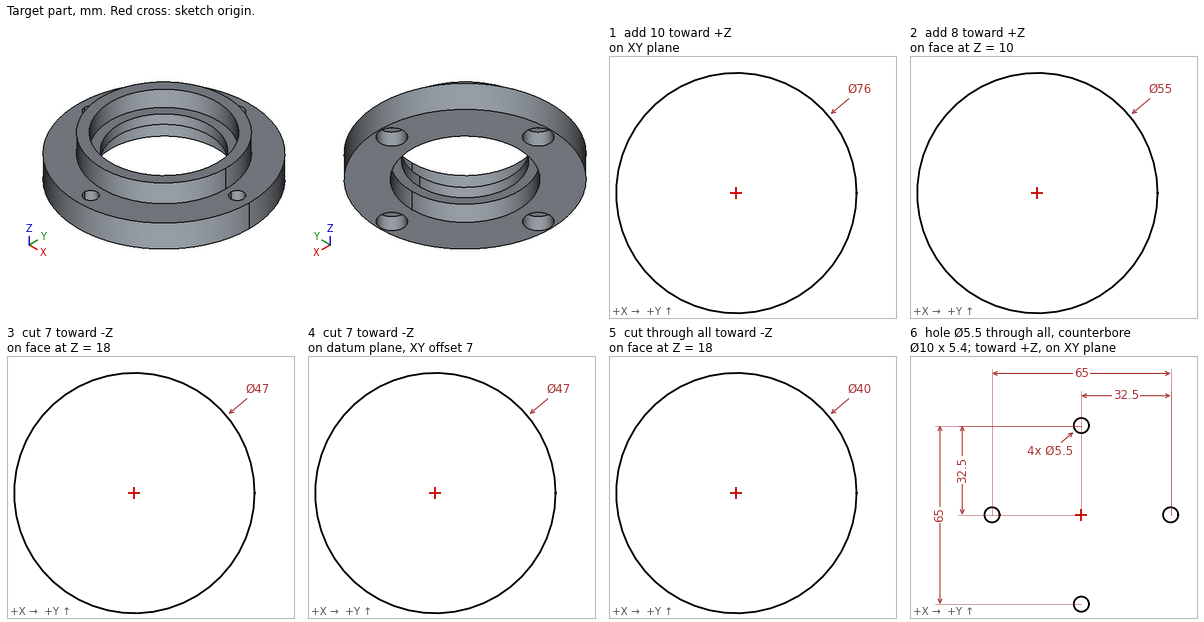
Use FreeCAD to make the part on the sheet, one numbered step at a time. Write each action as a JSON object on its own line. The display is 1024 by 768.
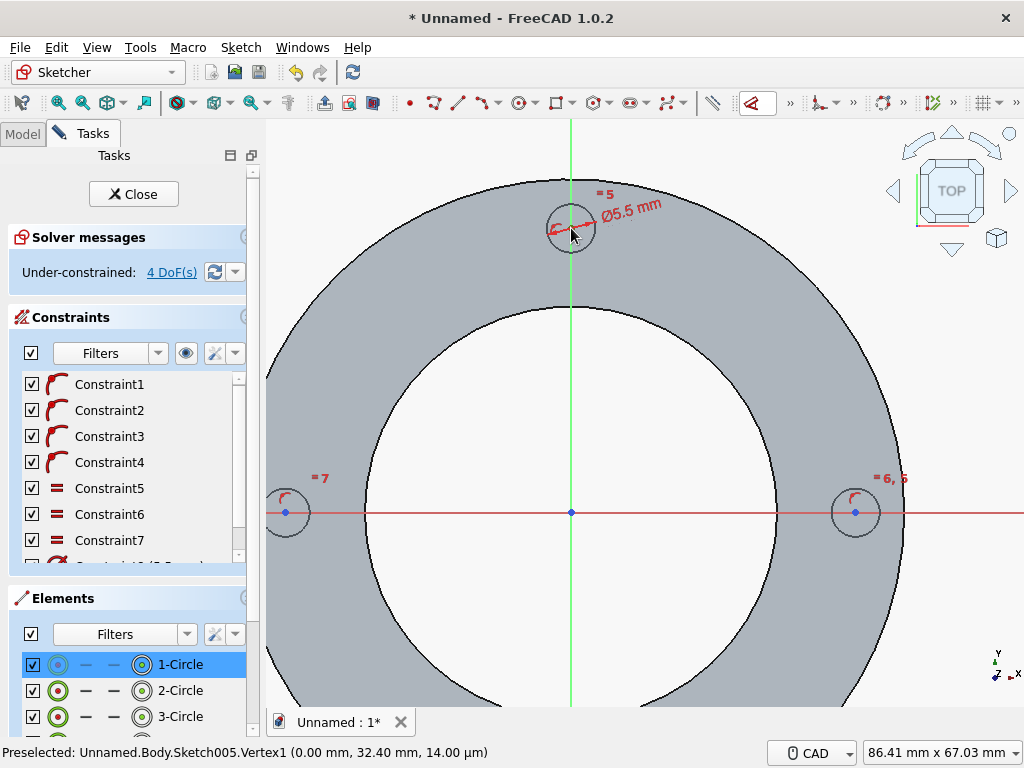
{"action": "scroll", "coordinate": [588, 210], "scroll_direction": "down", "scroll_amount": 2}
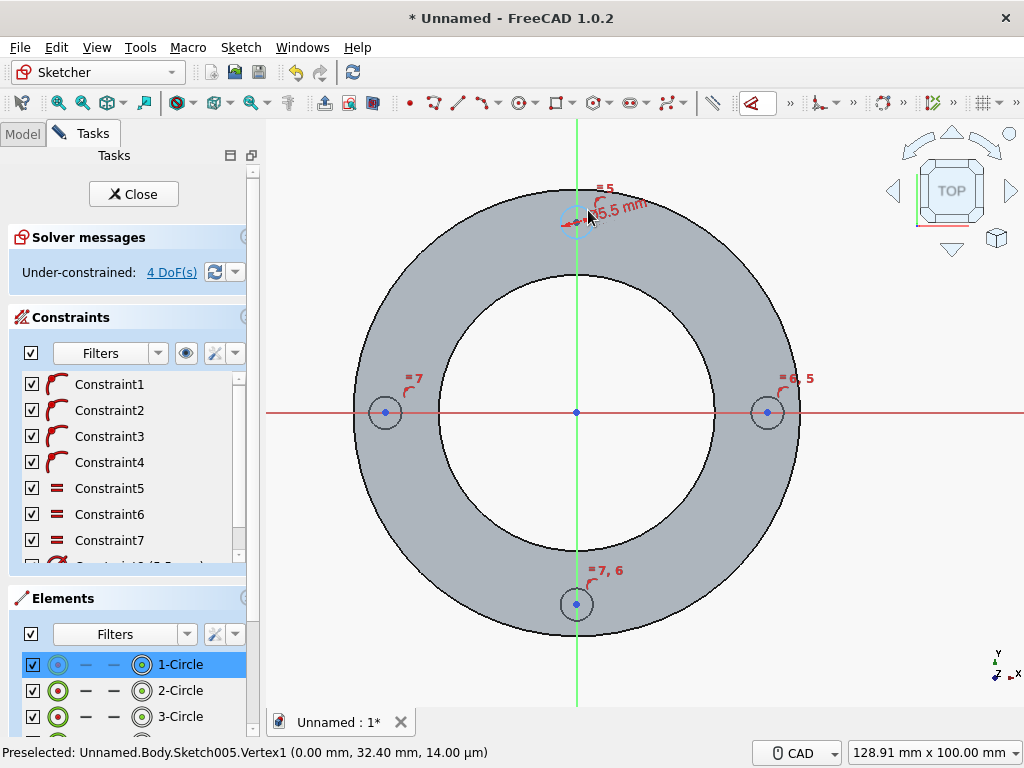
{"action": "left_click", "coordinate": [577, 605]}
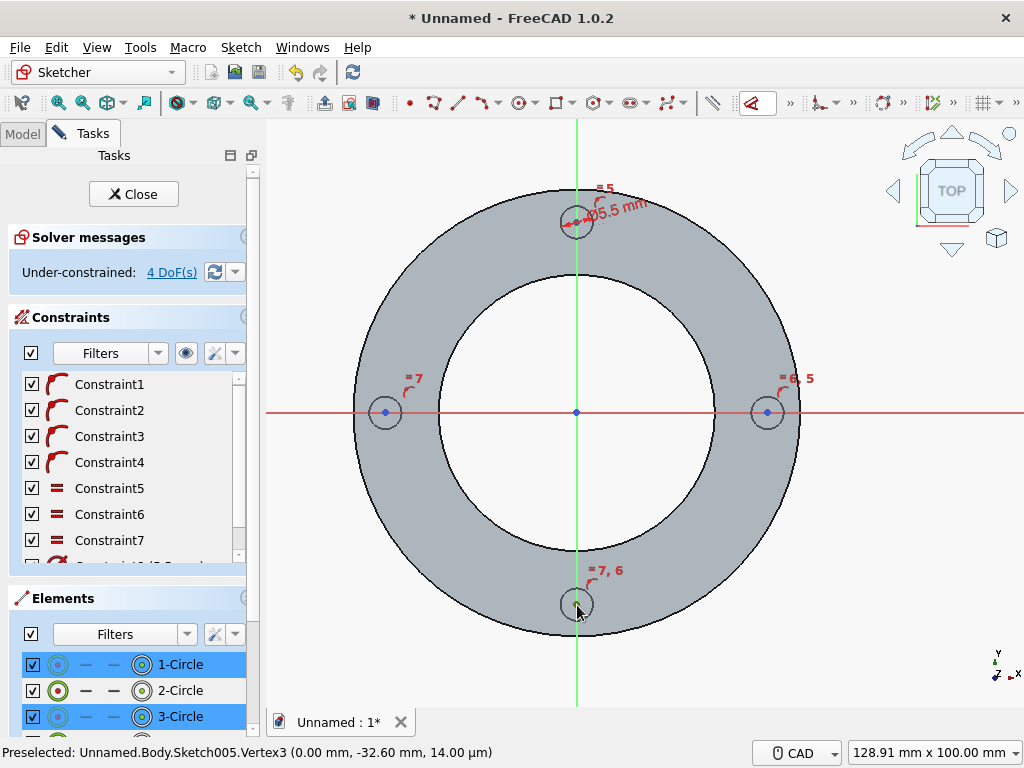
{"action": "left_click", "coordinate": [770, 104]}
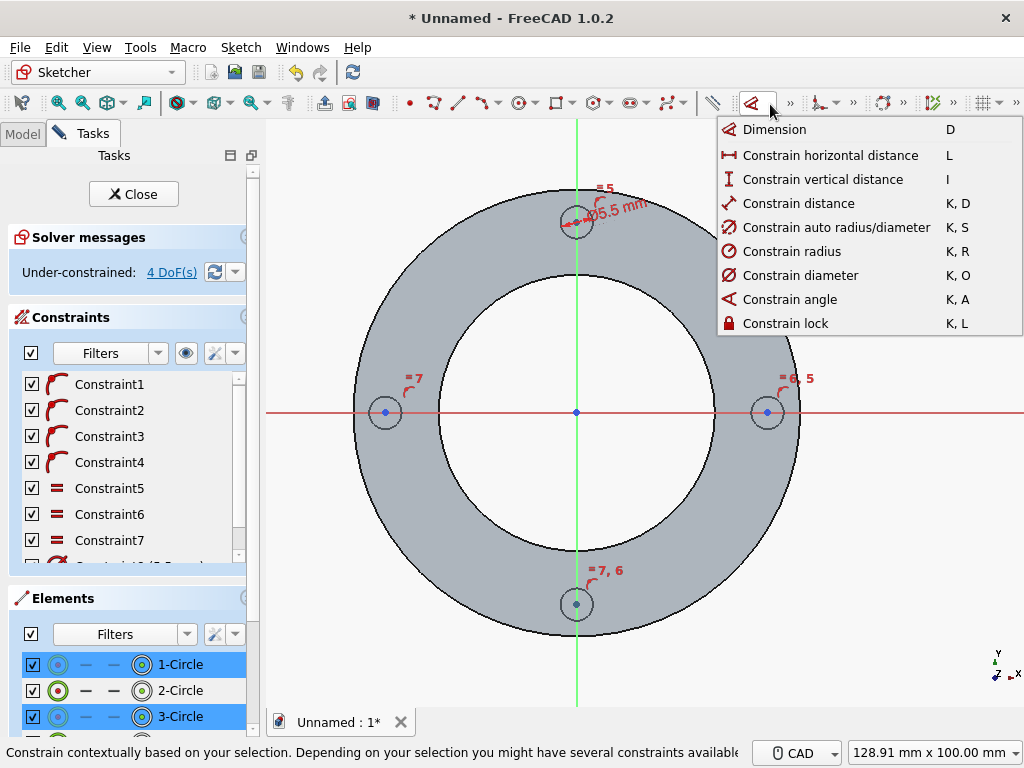
{"action": "left_click", "coordinate": [870, 179]}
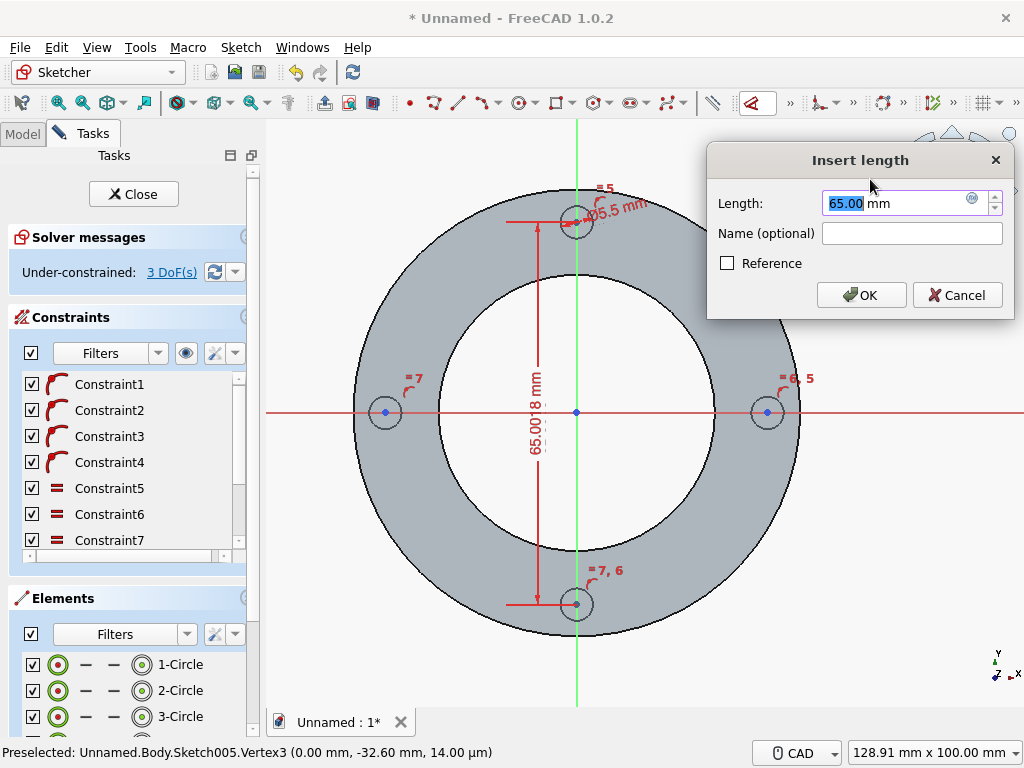
{"action": "type", "text": "65"}
{"action": "key", "text": "Return"}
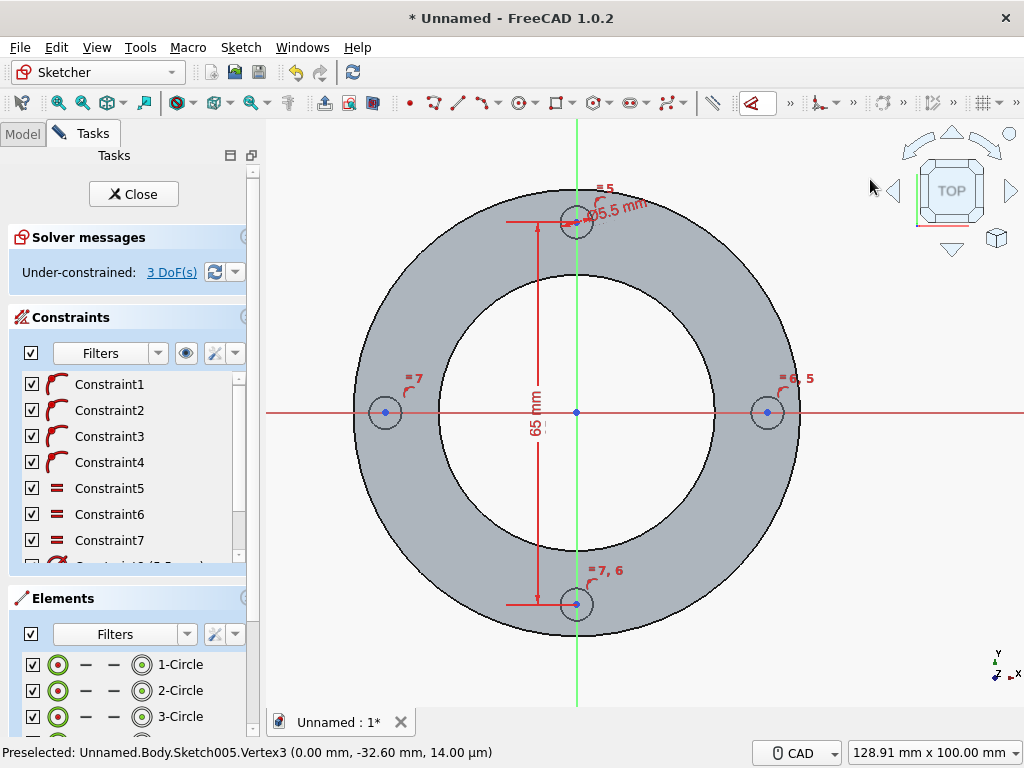
{"action": "left_click", "coordinate": [768, 413]}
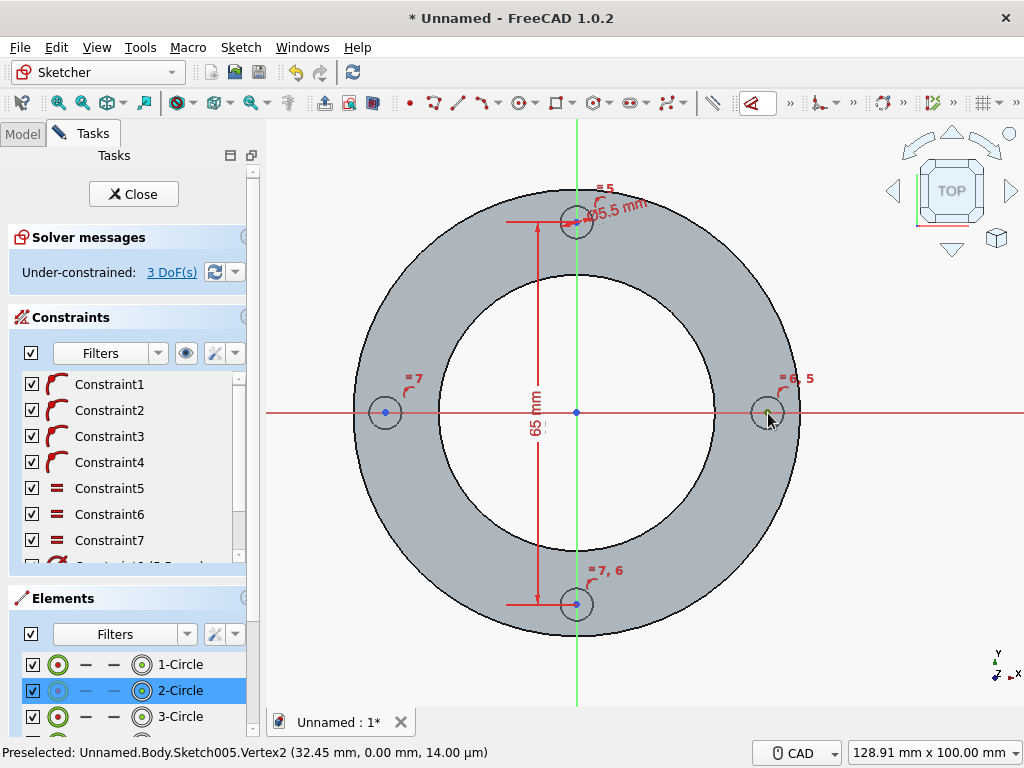
{"action": "left_click", "coordinate": [385, 413]}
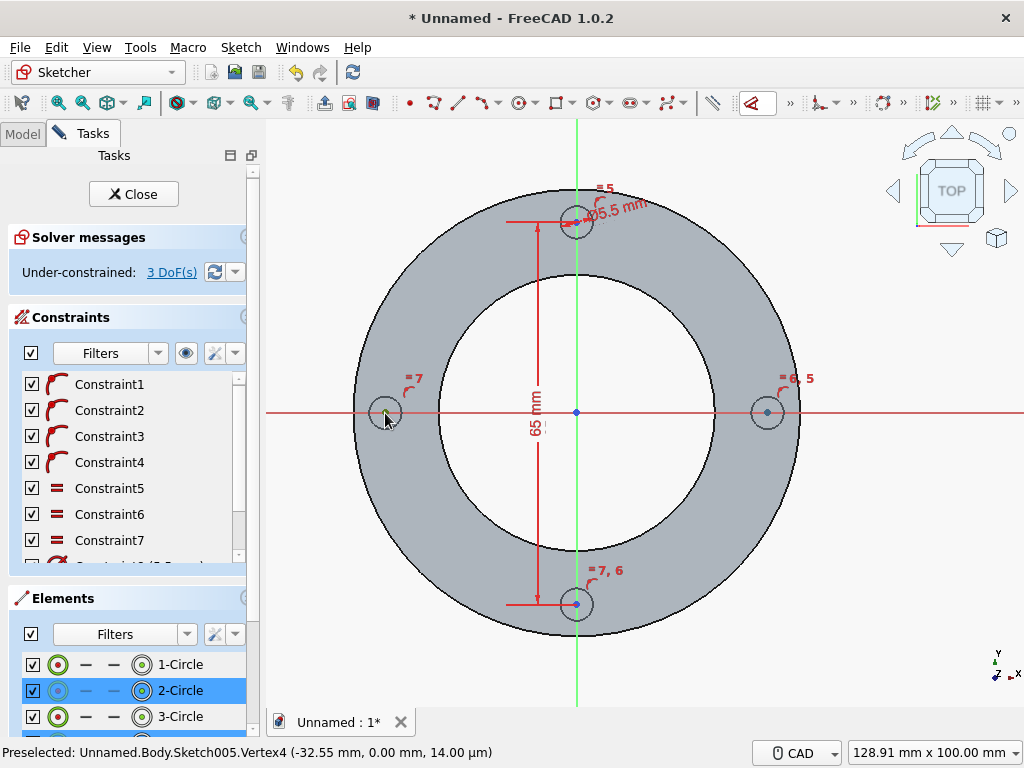
{"action": "key", "text": "l"}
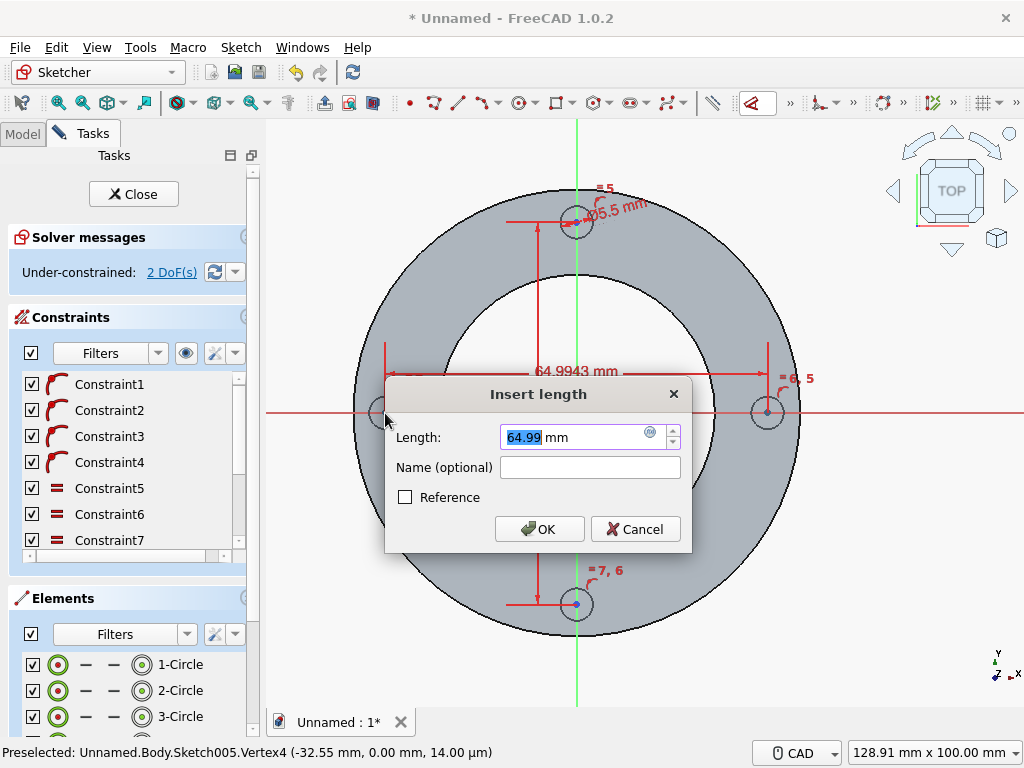
{"action": "type", "text": "65"}
{"action": "key", "text": "Return"}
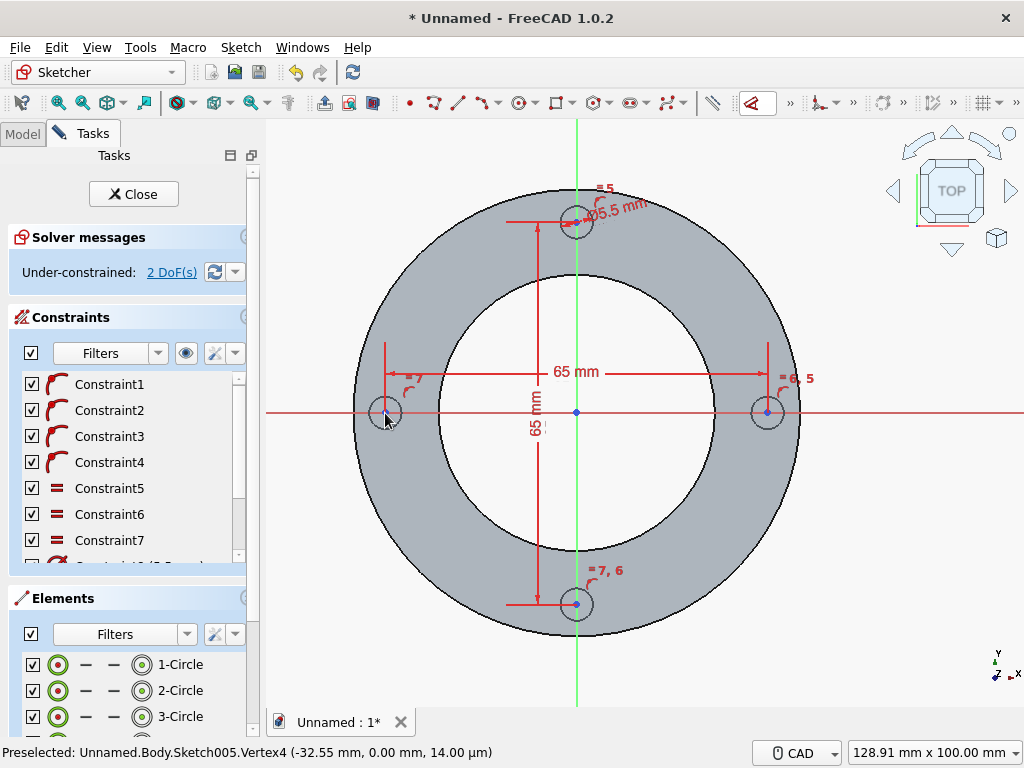
{"action": "left_click", "coordinate": [577, 222]}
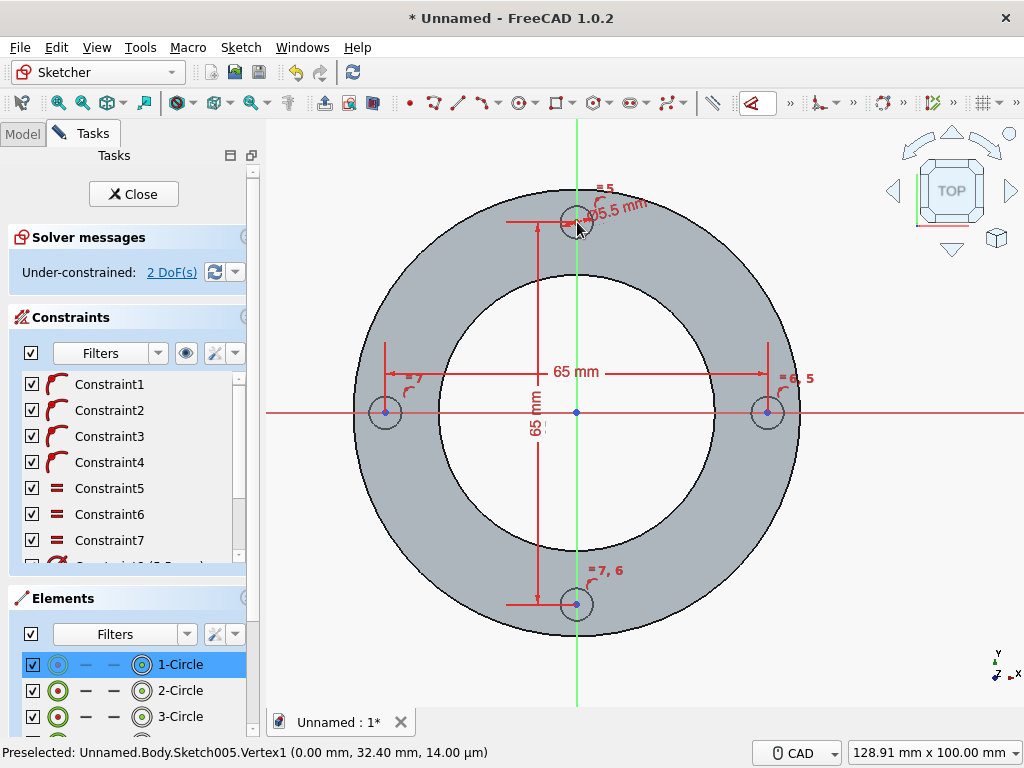
{"action": "key", "text": "i"}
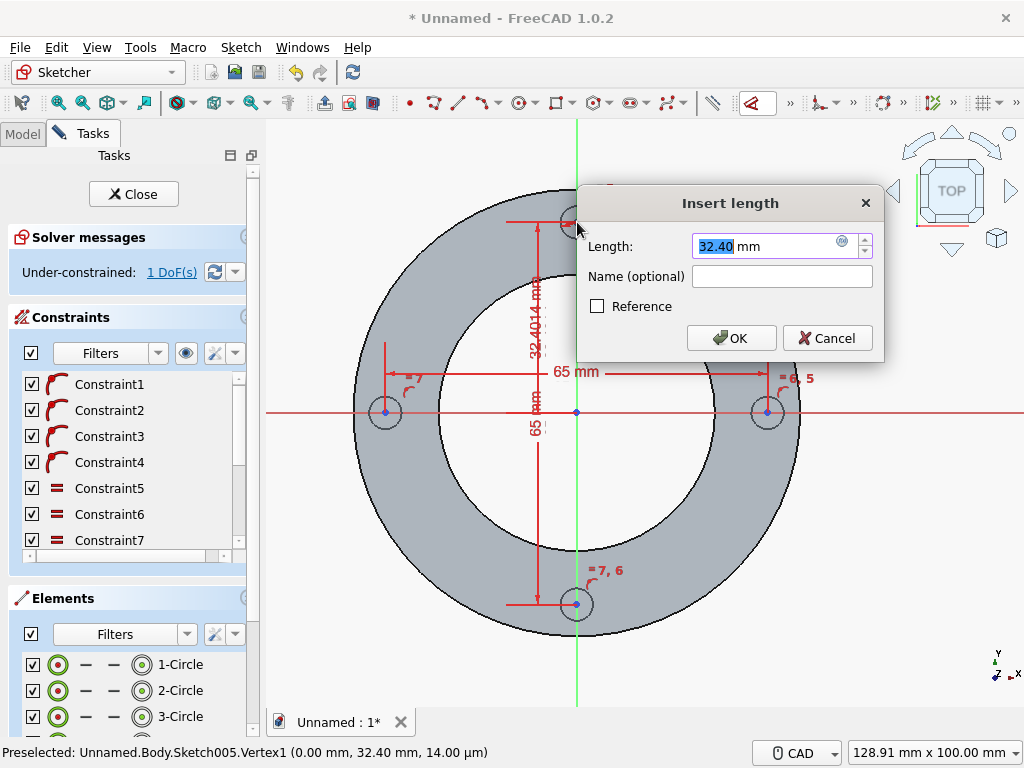
{"action": "type", "text": "32.5"}
{"action": "key", "text": "Return"}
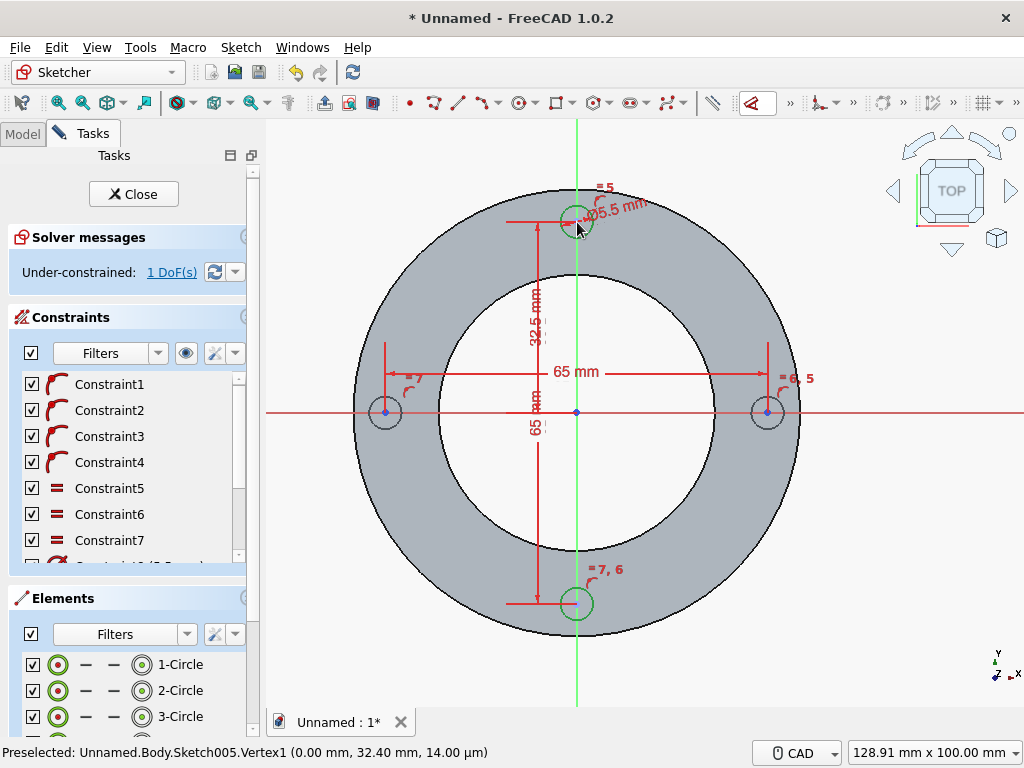
{"action": "left_click", "coordinate": [768, 413]}